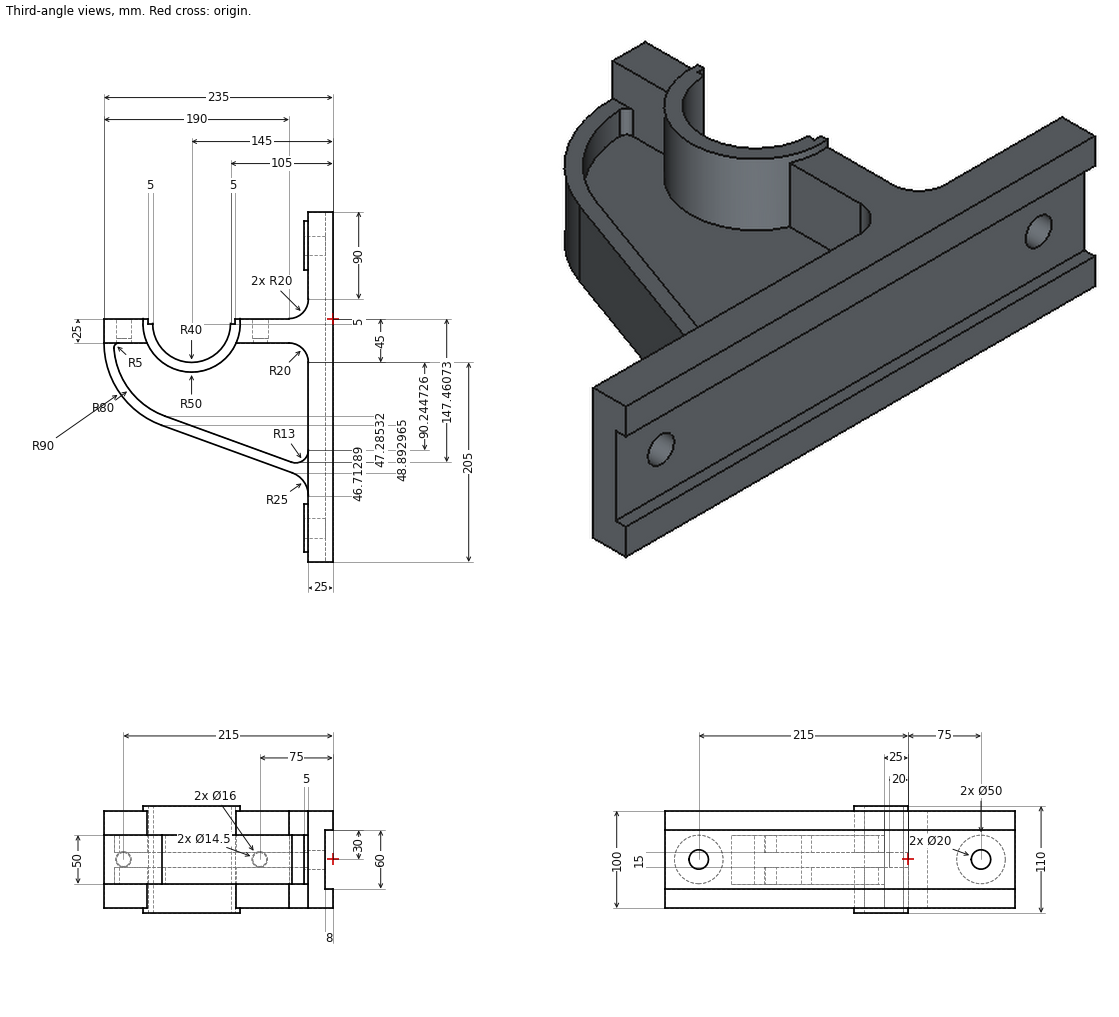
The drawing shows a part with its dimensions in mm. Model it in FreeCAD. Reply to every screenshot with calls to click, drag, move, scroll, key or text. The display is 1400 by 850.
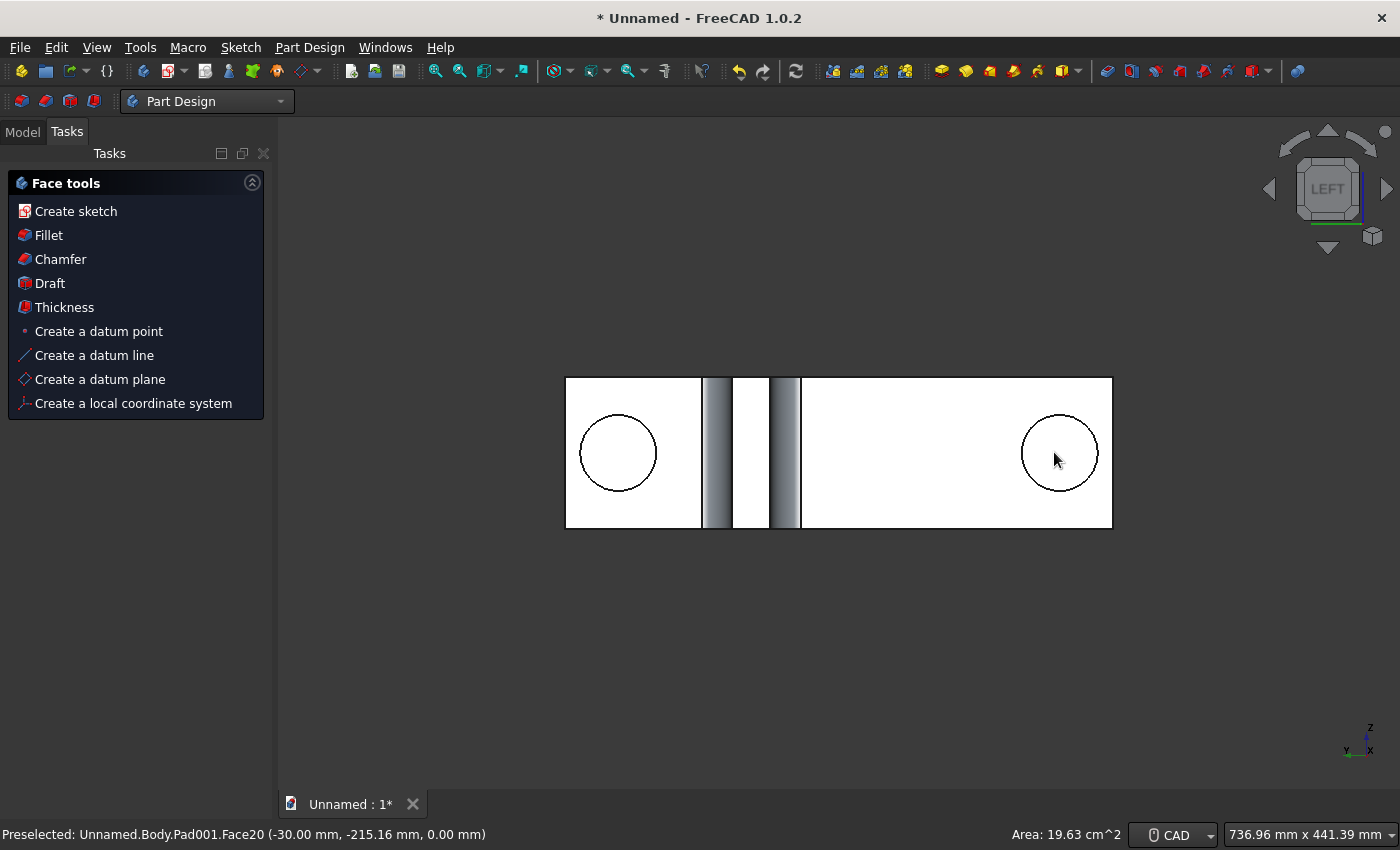
click(168, 72)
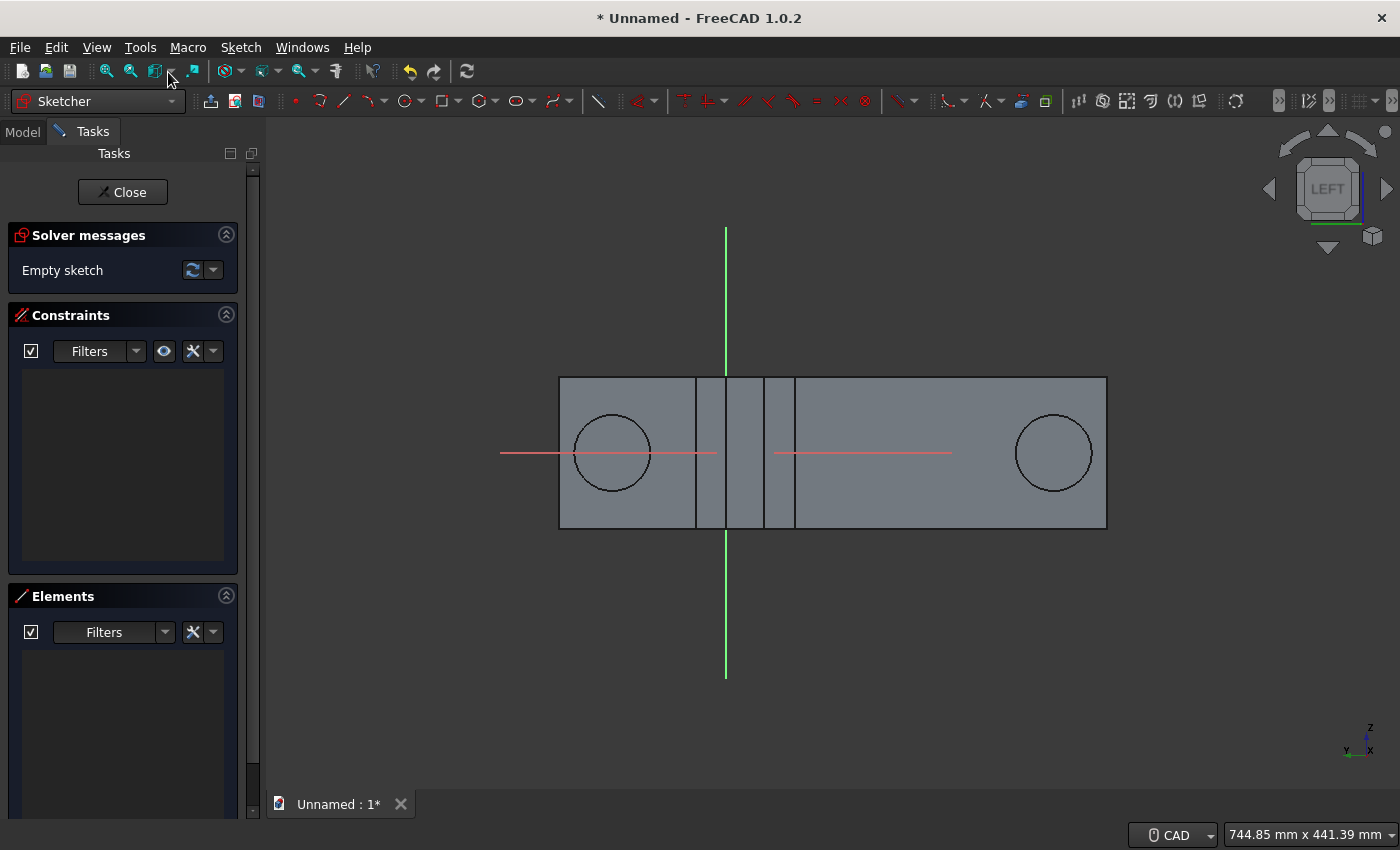
scroll(972, 453, up, 2)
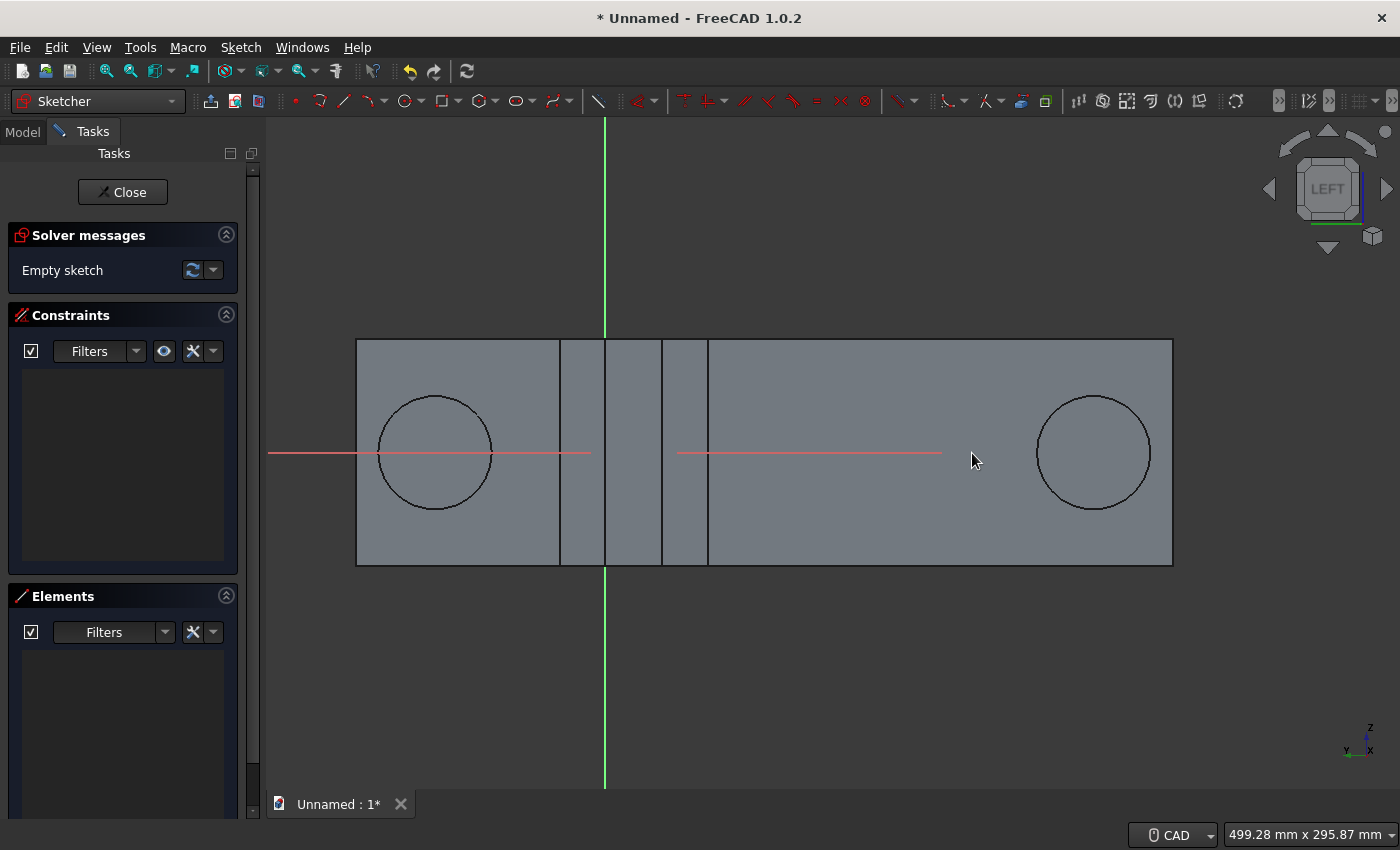
click(406, 102)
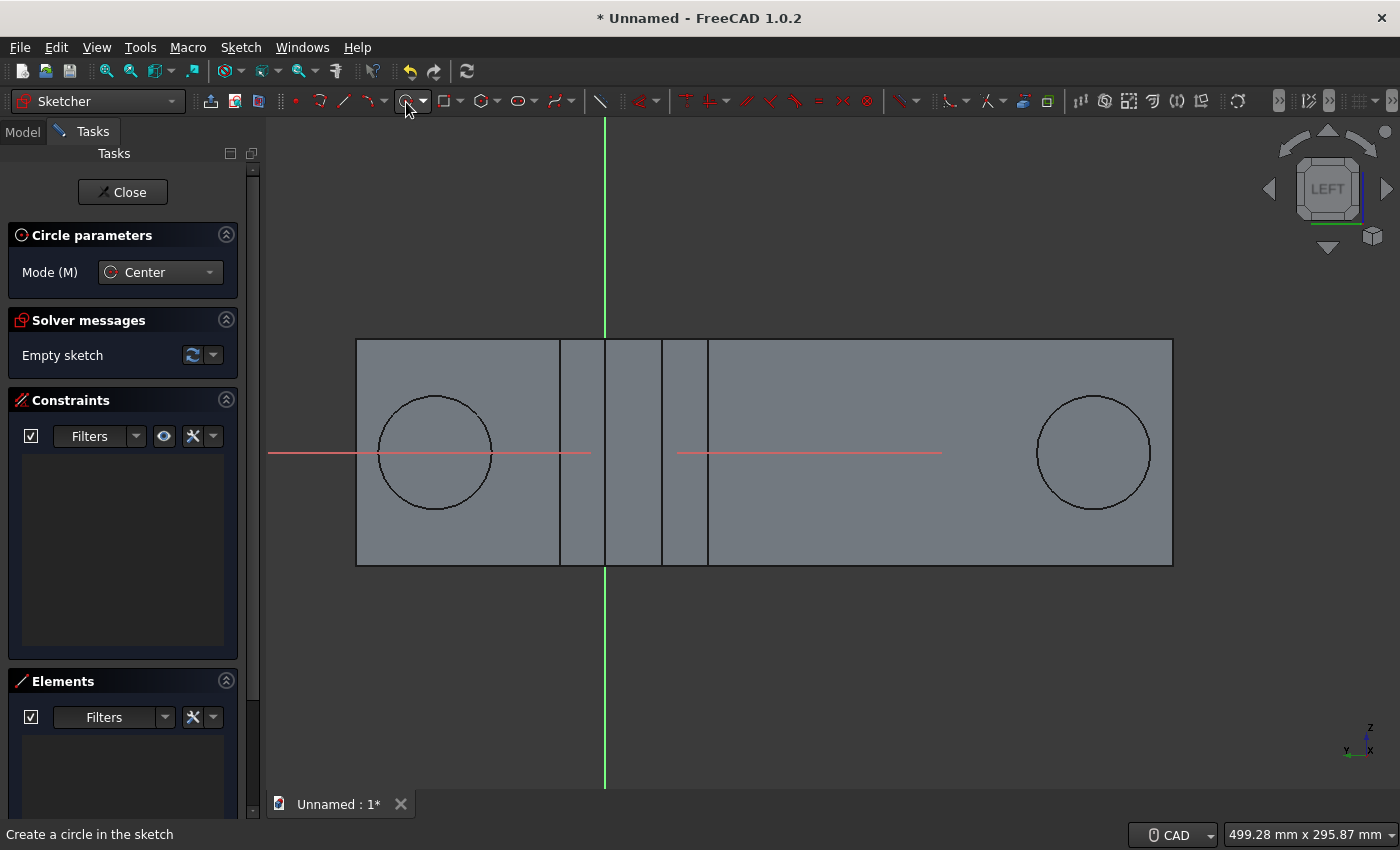
click(435, 453)
move(451, 437)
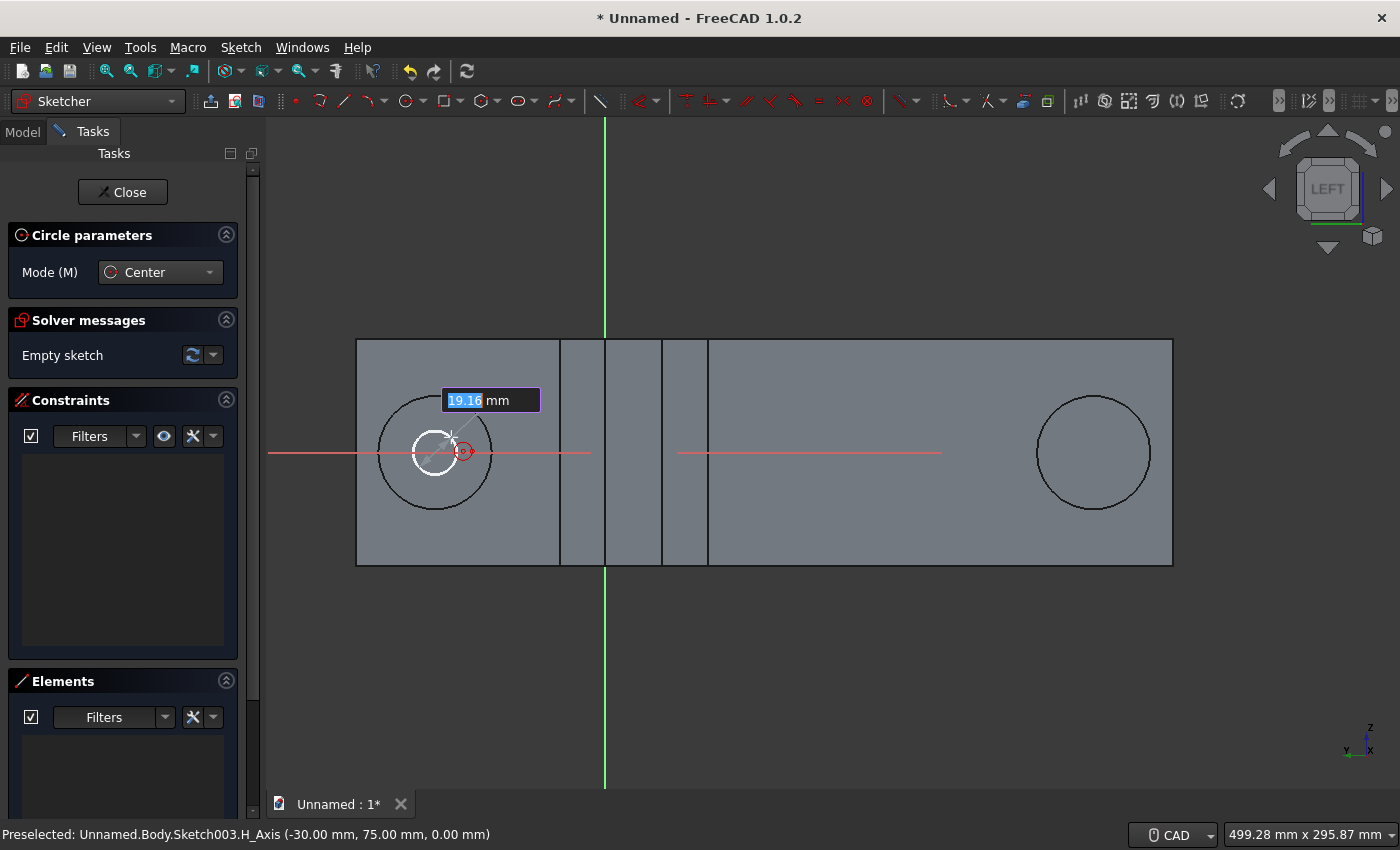
text(20)
key(Return)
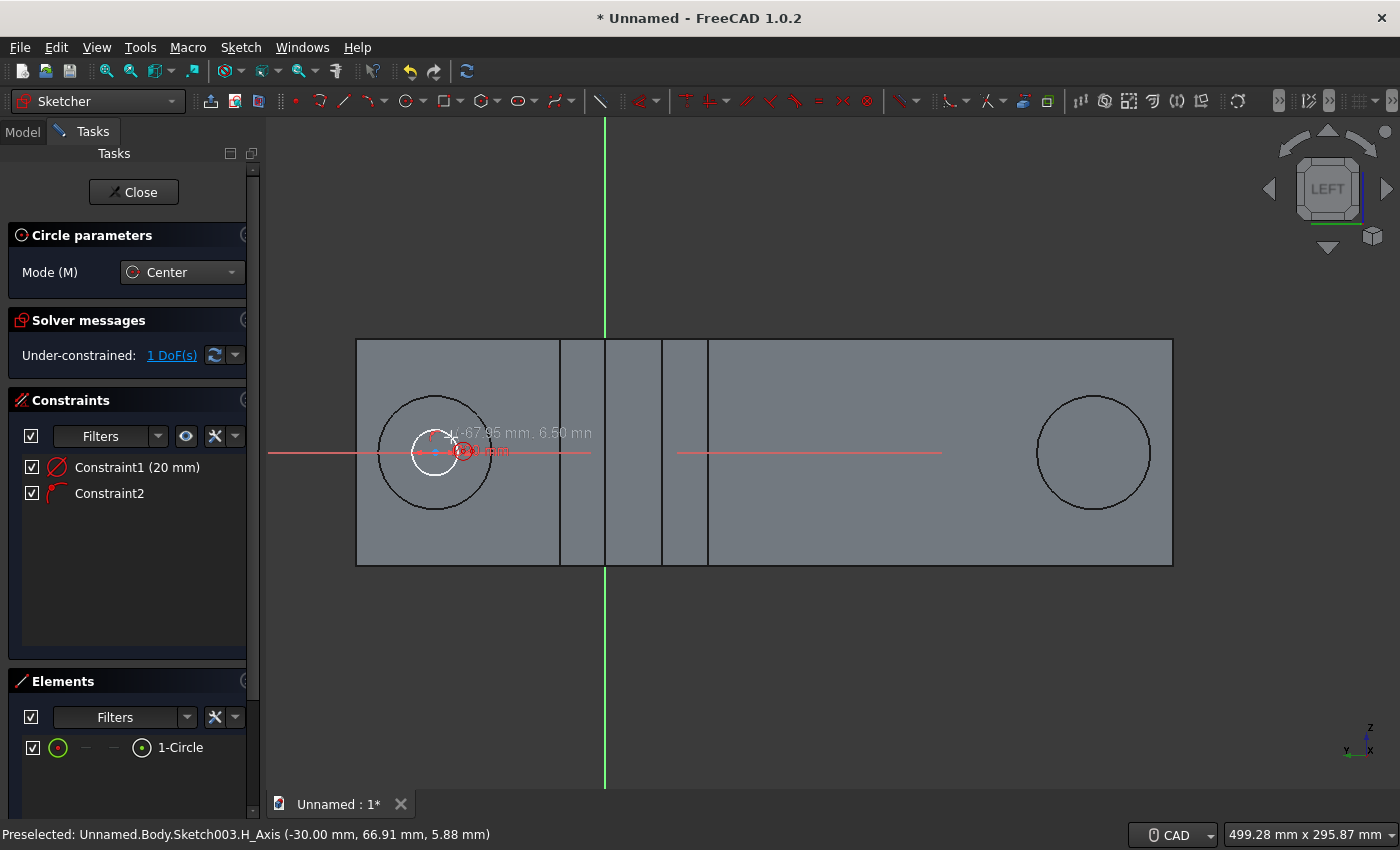
click(1094, 453)
move(1110, 437)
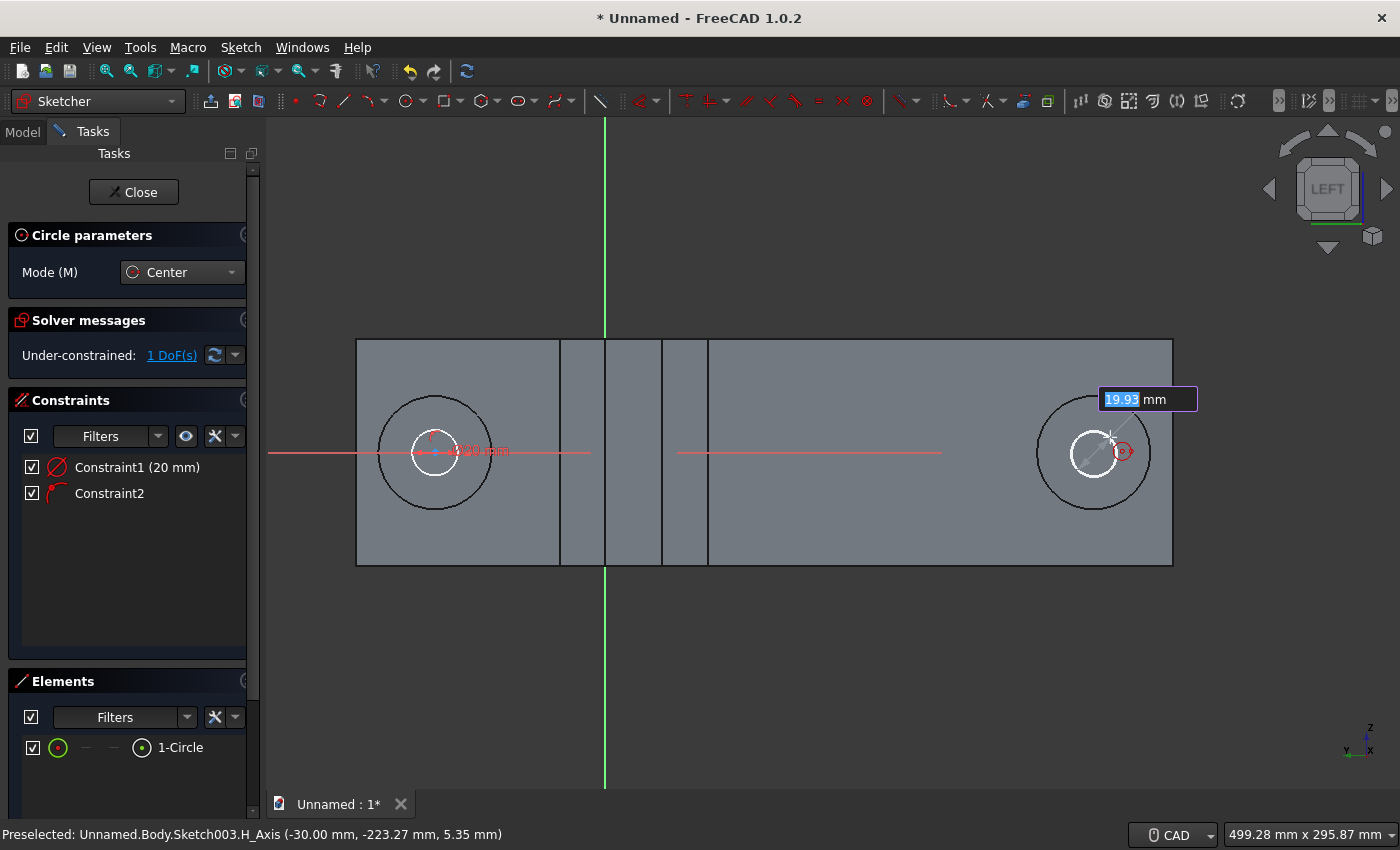
text(20)
key(Return)
key(Escape)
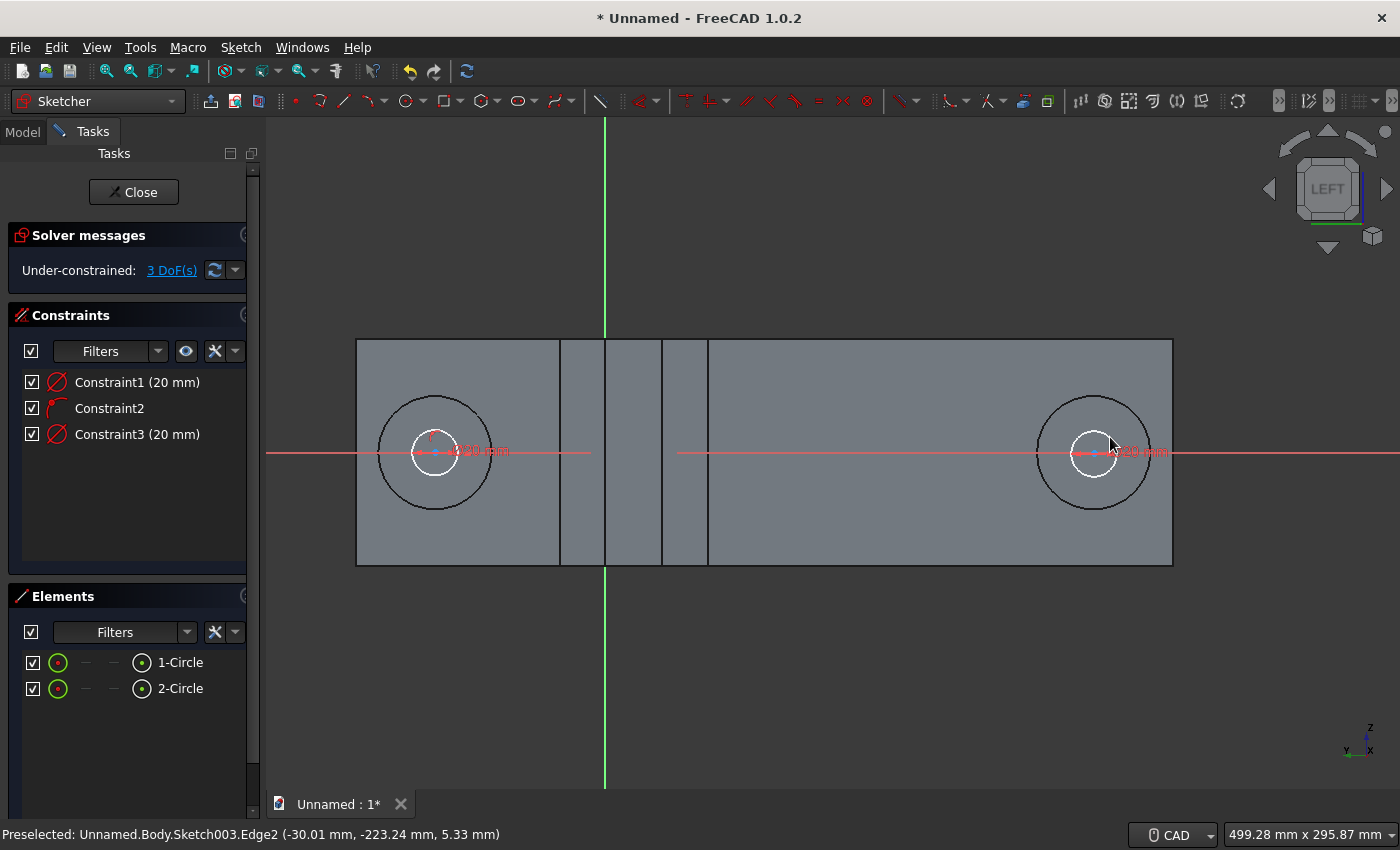
click(1094, 454)